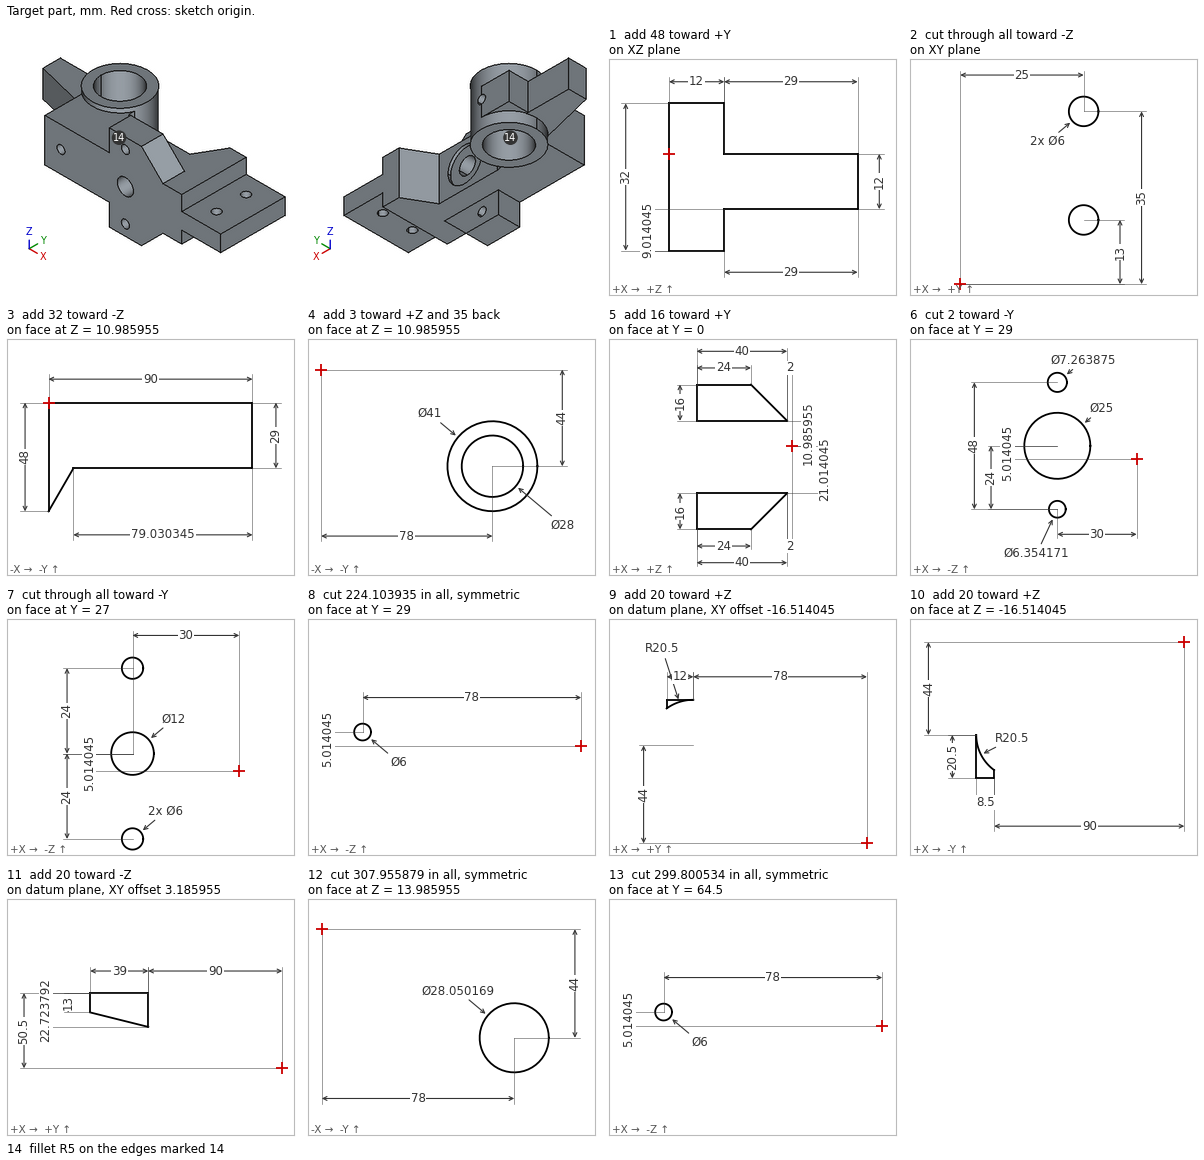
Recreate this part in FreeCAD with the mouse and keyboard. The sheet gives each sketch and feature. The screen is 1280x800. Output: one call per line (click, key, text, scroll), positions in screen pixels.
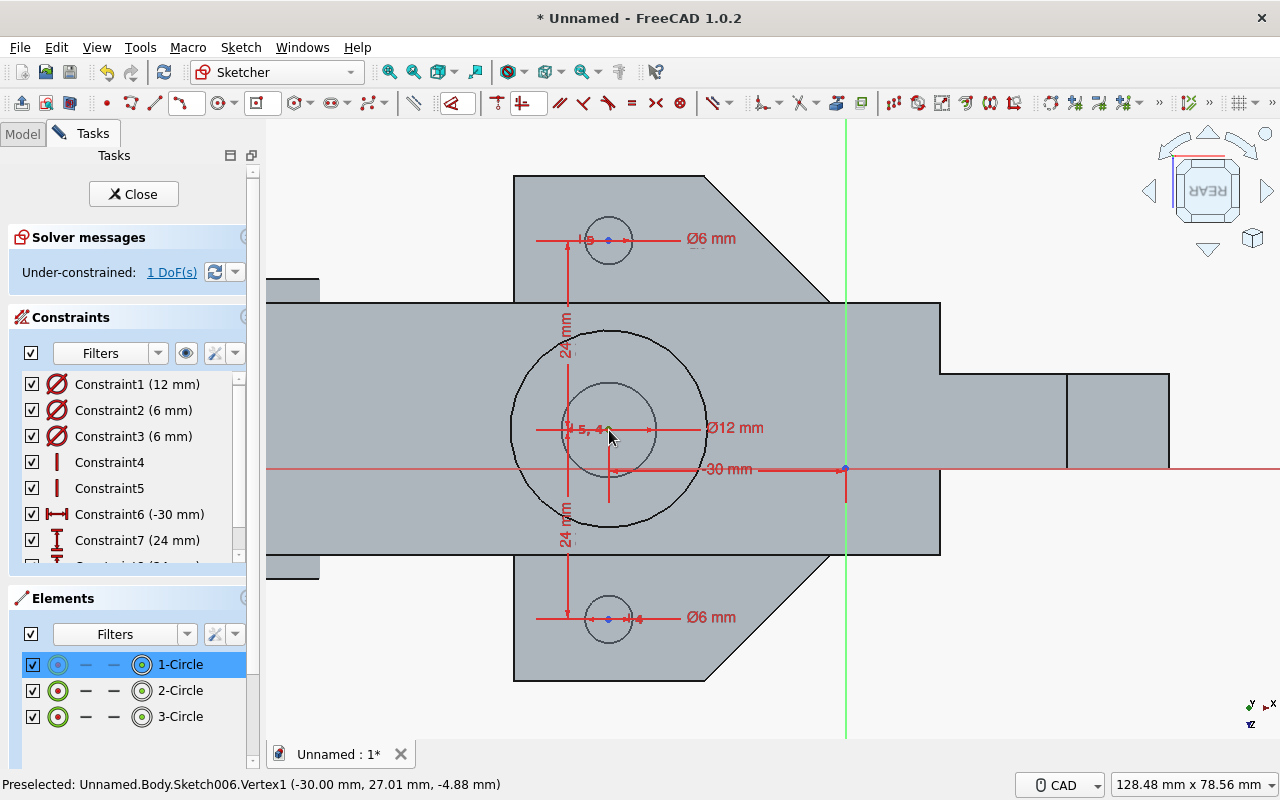
key(i)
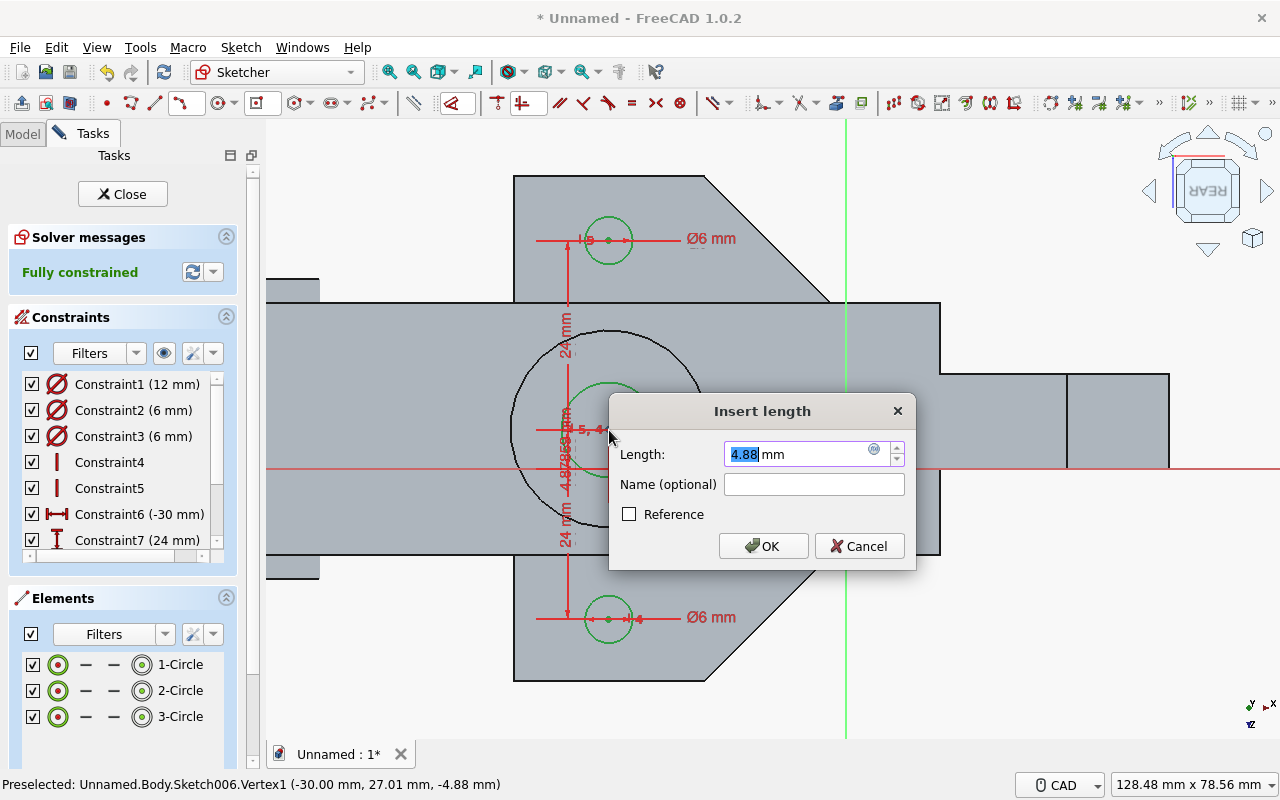
text(5.014045)
key(Return)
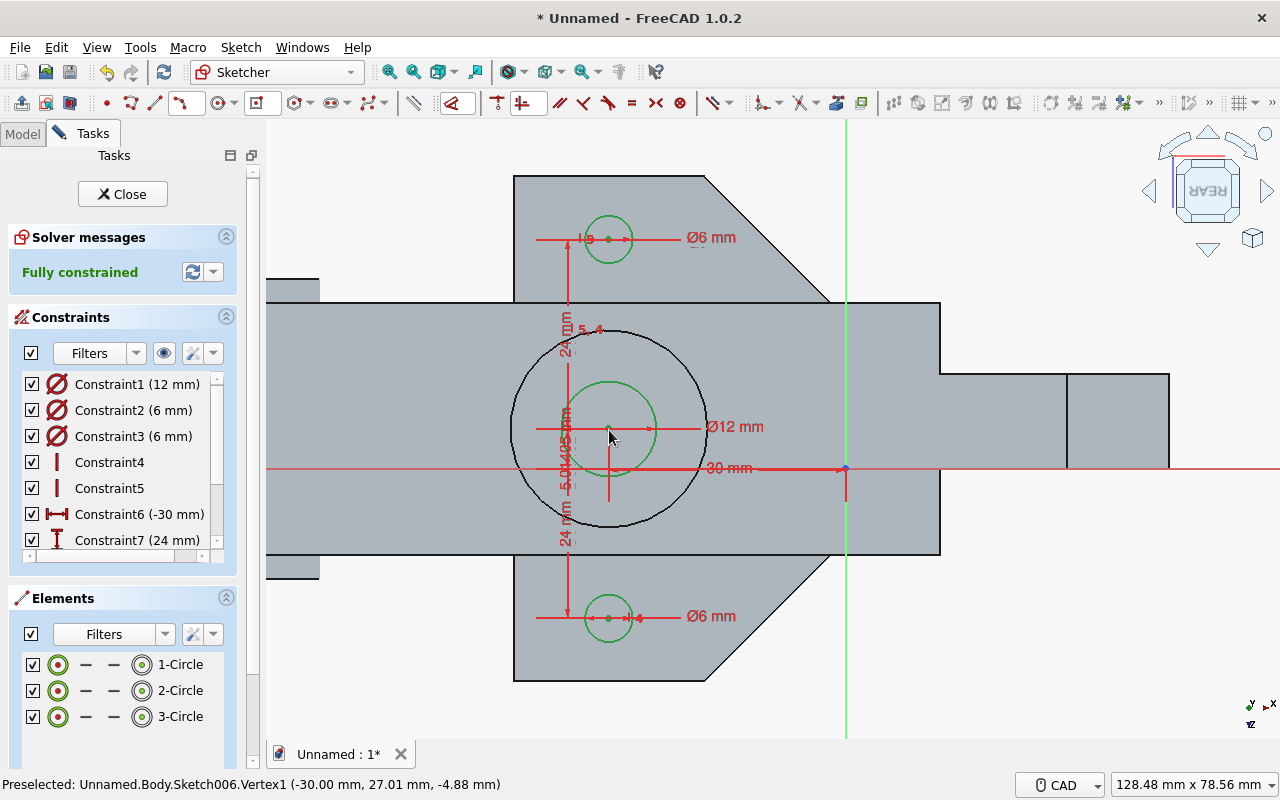
click(123, 194)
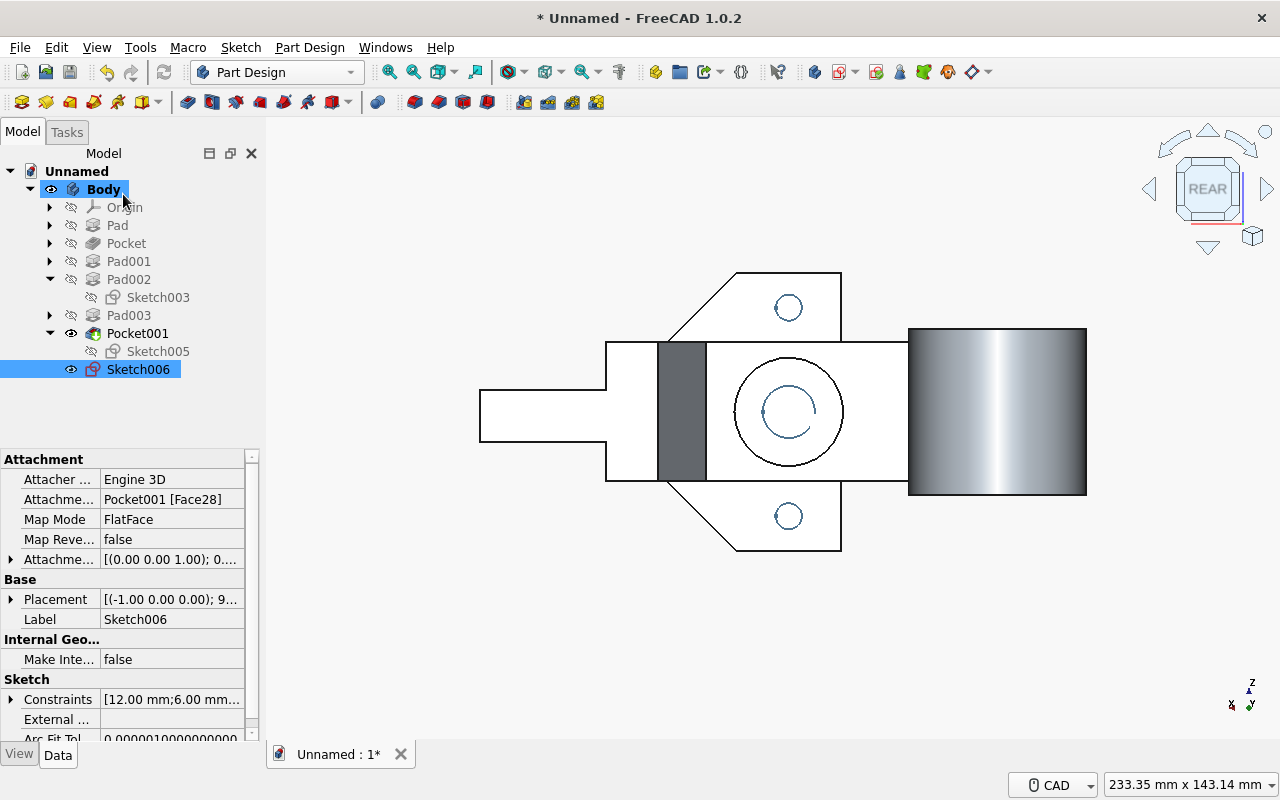
click(188, 102)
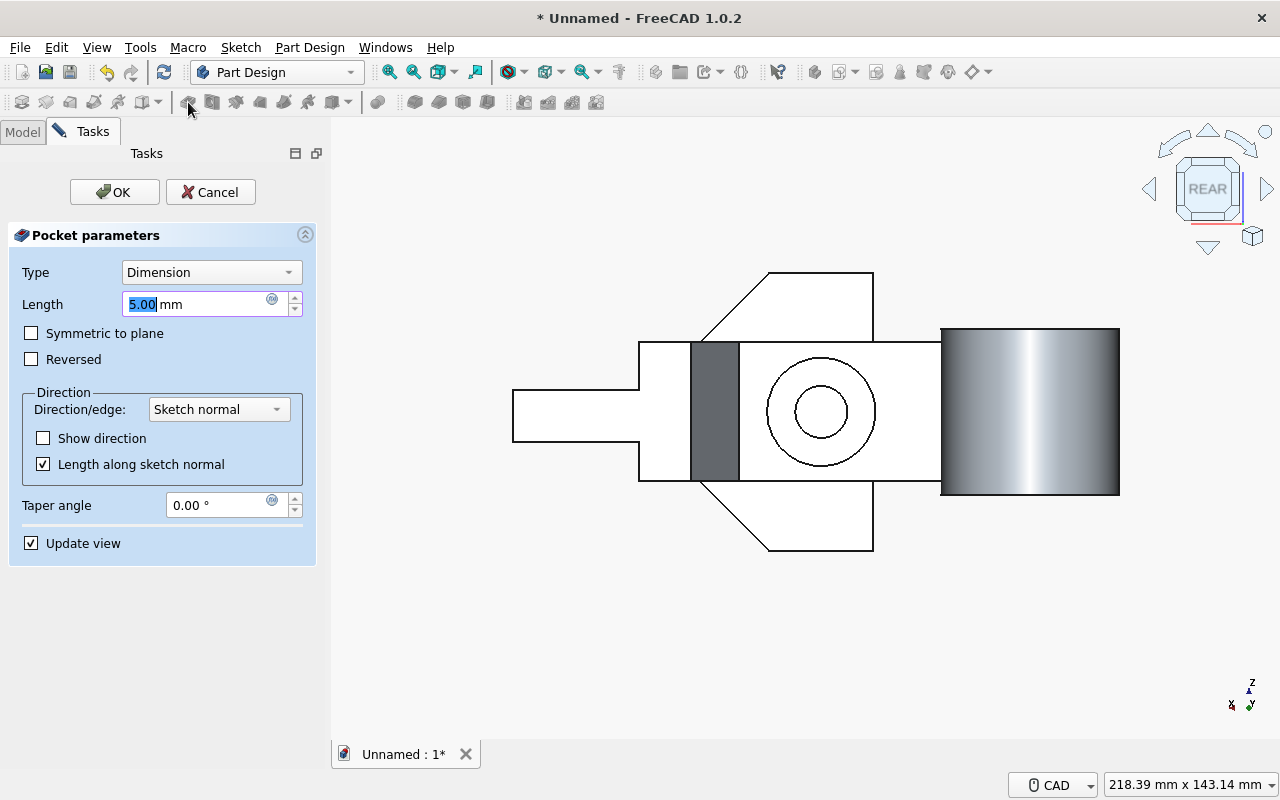
click(212, 272)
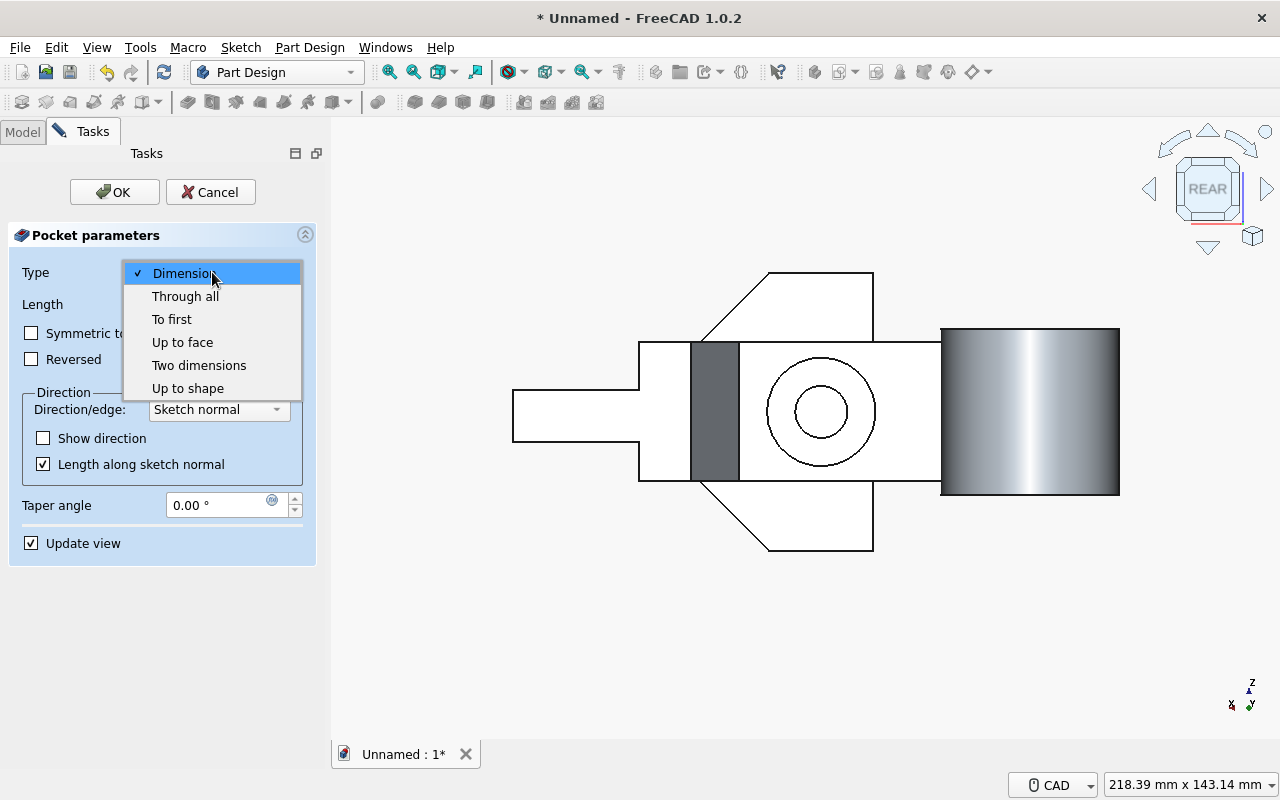
click(212, 296)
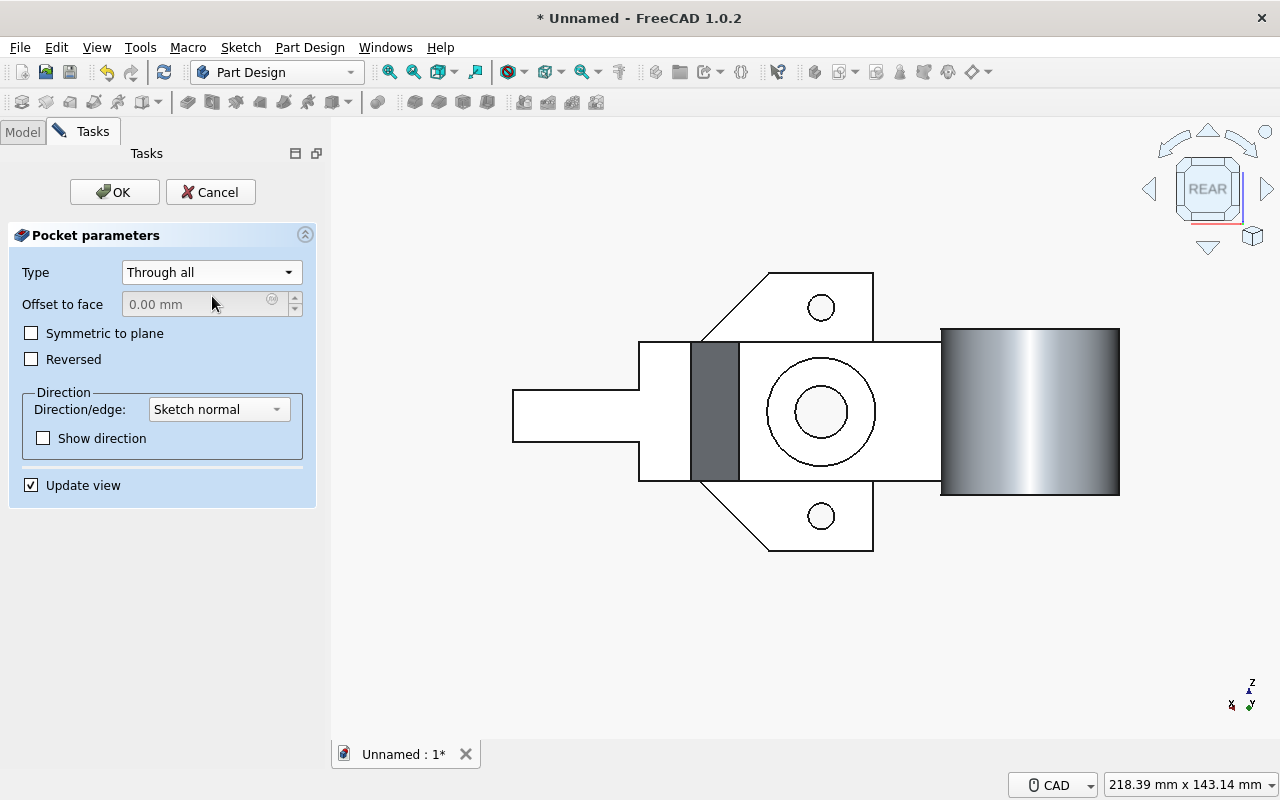
click(115, 192)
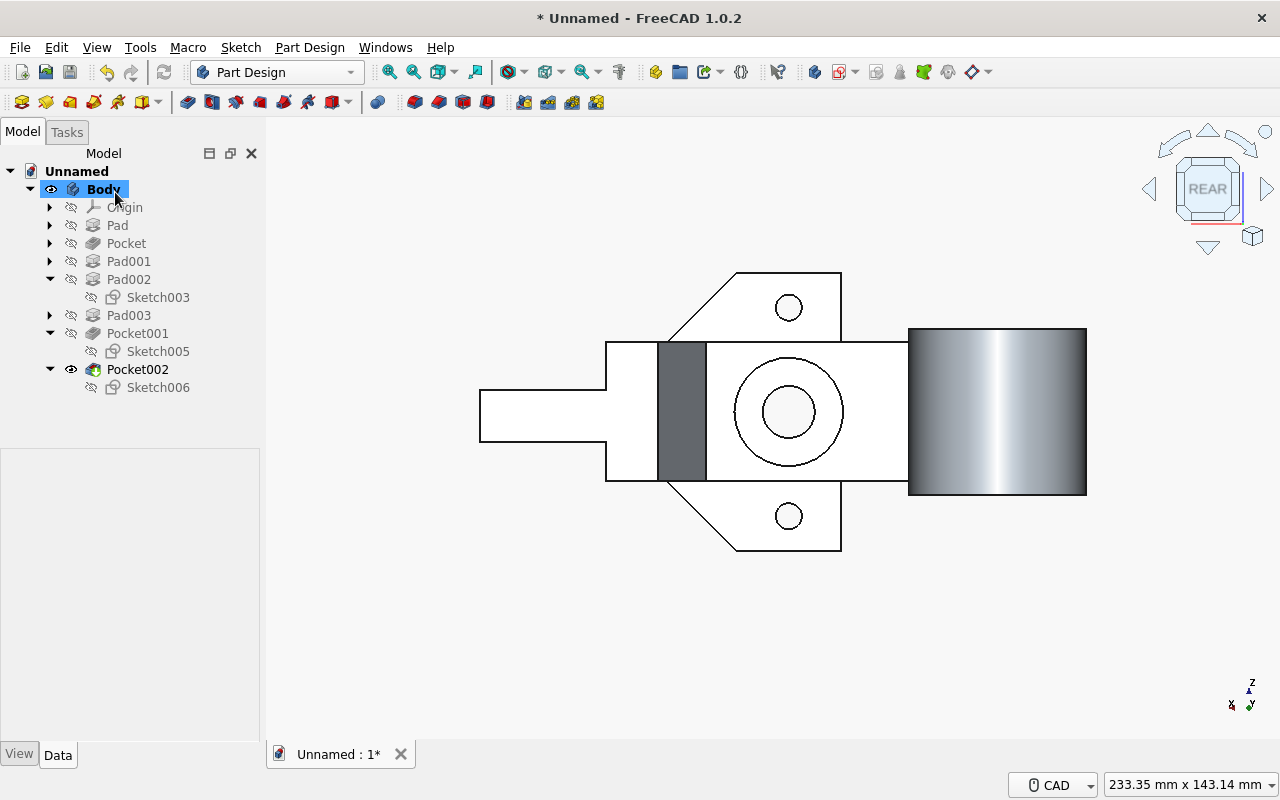
click(887, 431)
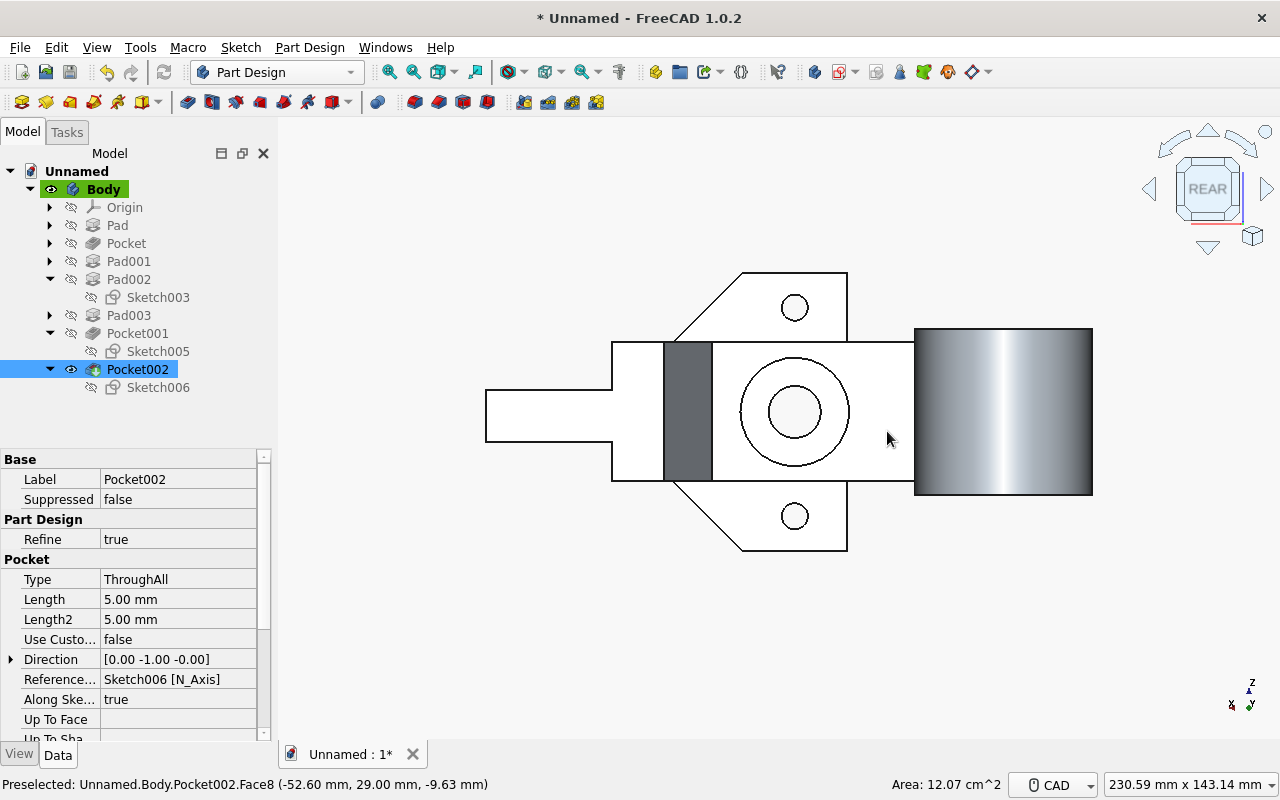
click(840, 72)